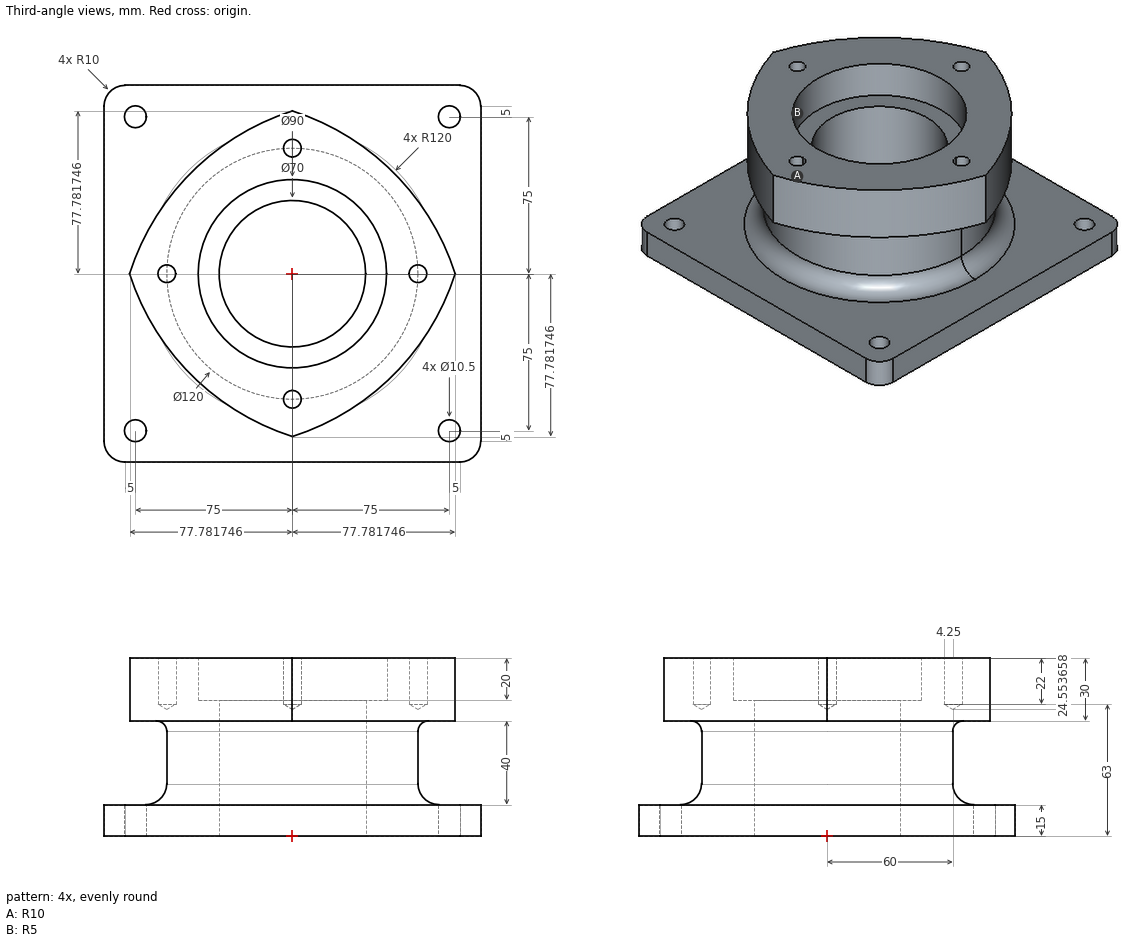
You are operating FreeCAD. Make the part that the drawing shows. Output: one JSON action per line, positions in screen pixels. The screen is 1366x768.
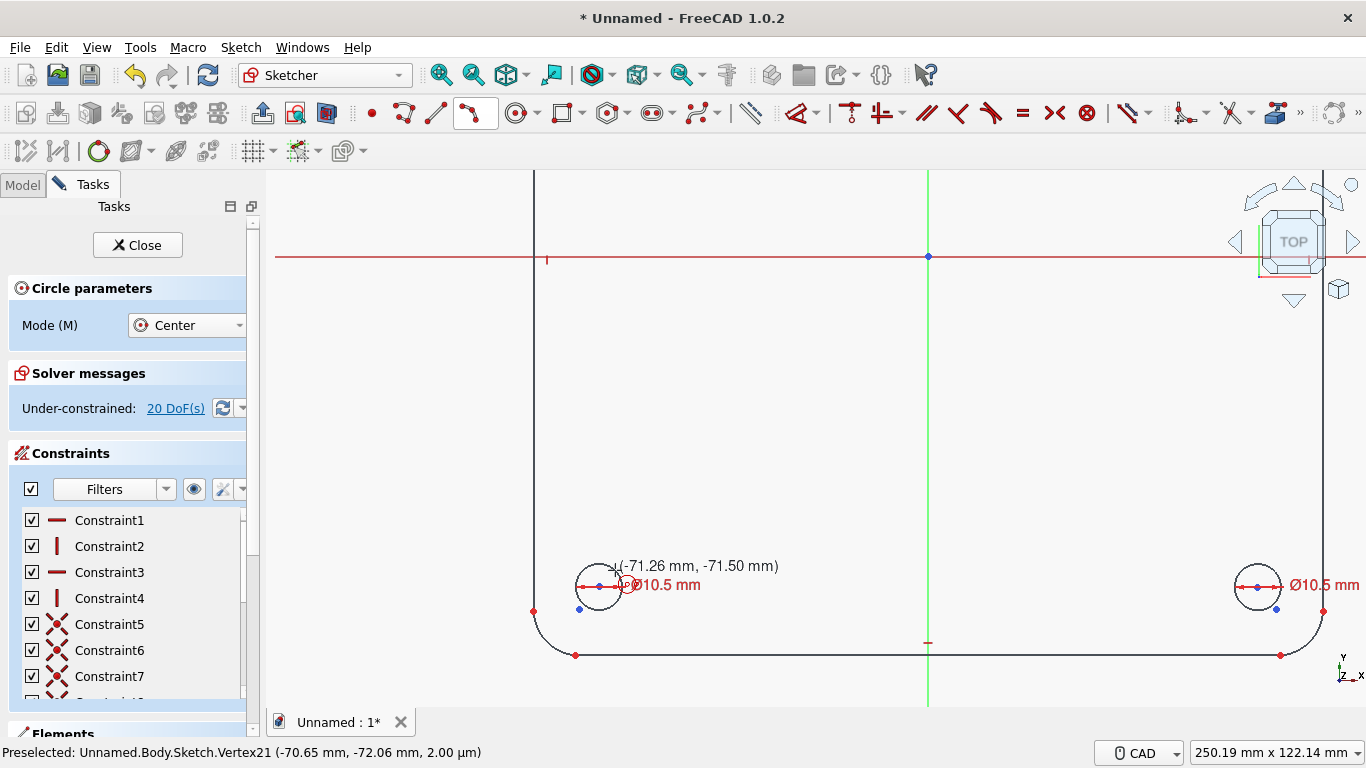
{"action": "scroll", "coordinate": [600, 587], "scroll_direction": "down", "scroll_amount": 4}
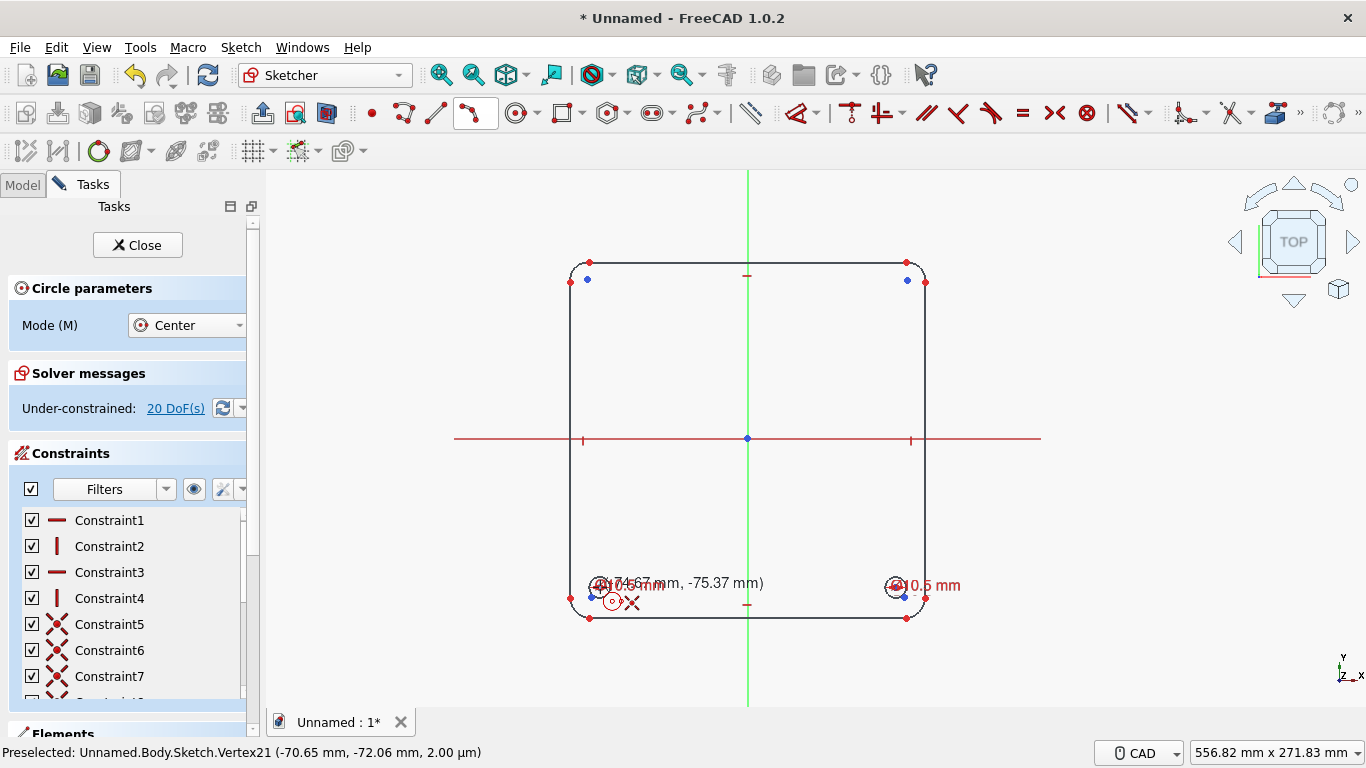
{"action": "scroll", "coordinate": [896, 291], "scroll_direction": "up", "scroll_amount": 4}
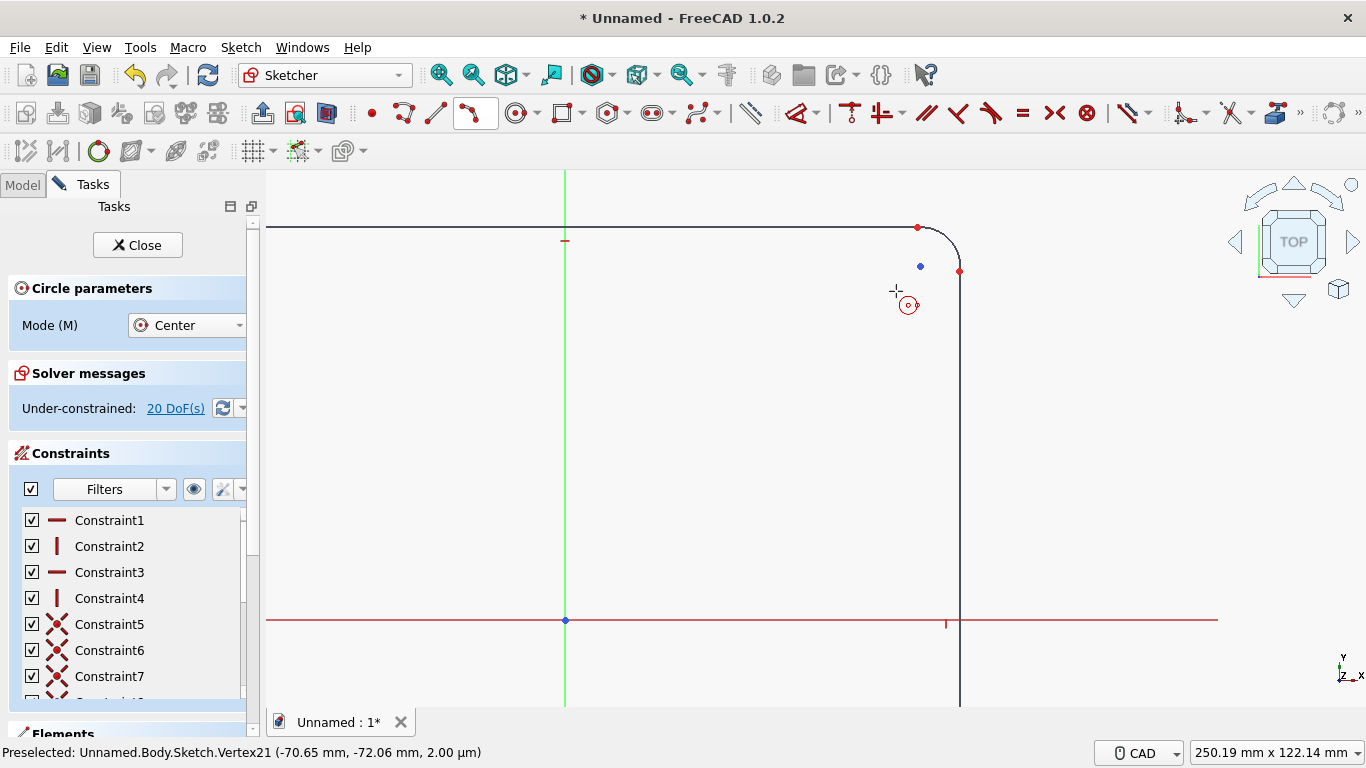
{"action": "left_click", "coordinate": [895, 290]}
{"action": "mouse_move", "coordinate": [879, 274]}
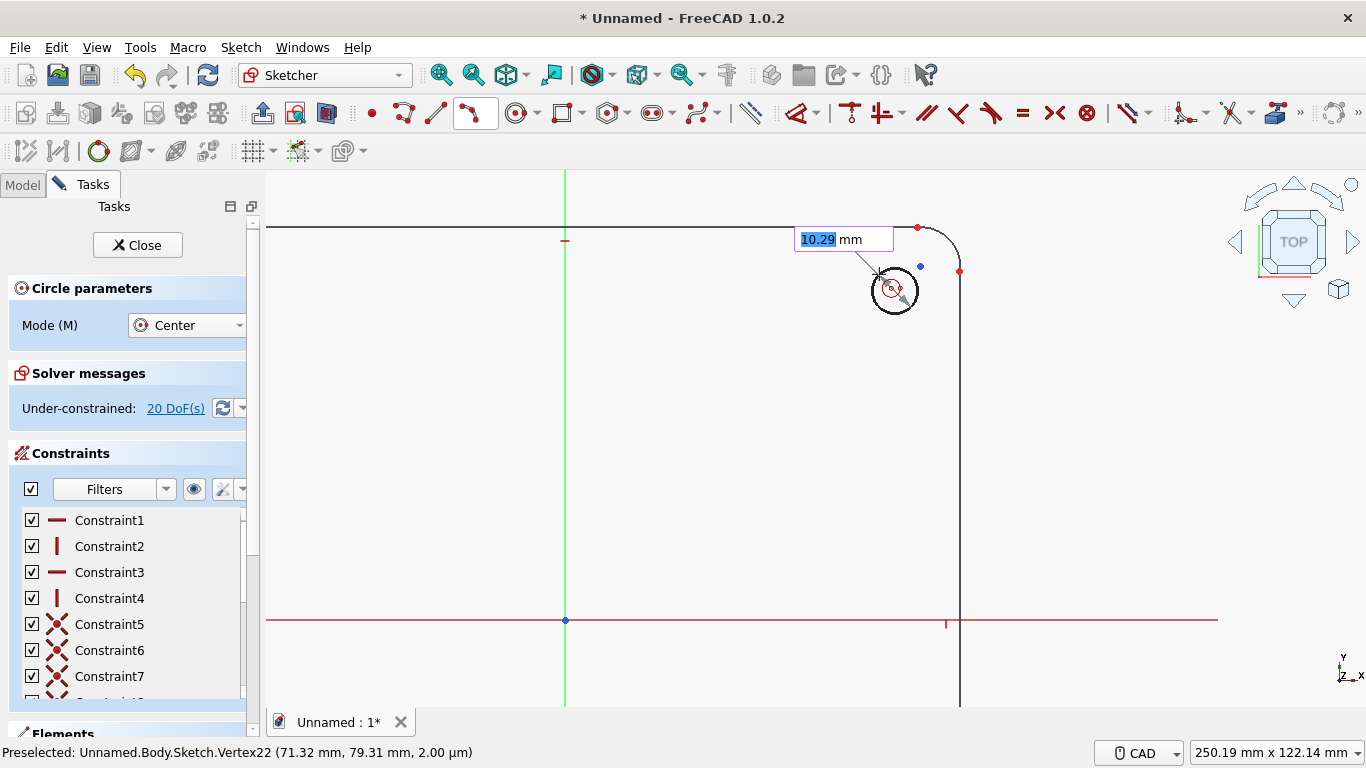
{"action": "type", "text": "10.5"}
{"action": "key", "text": "Return"}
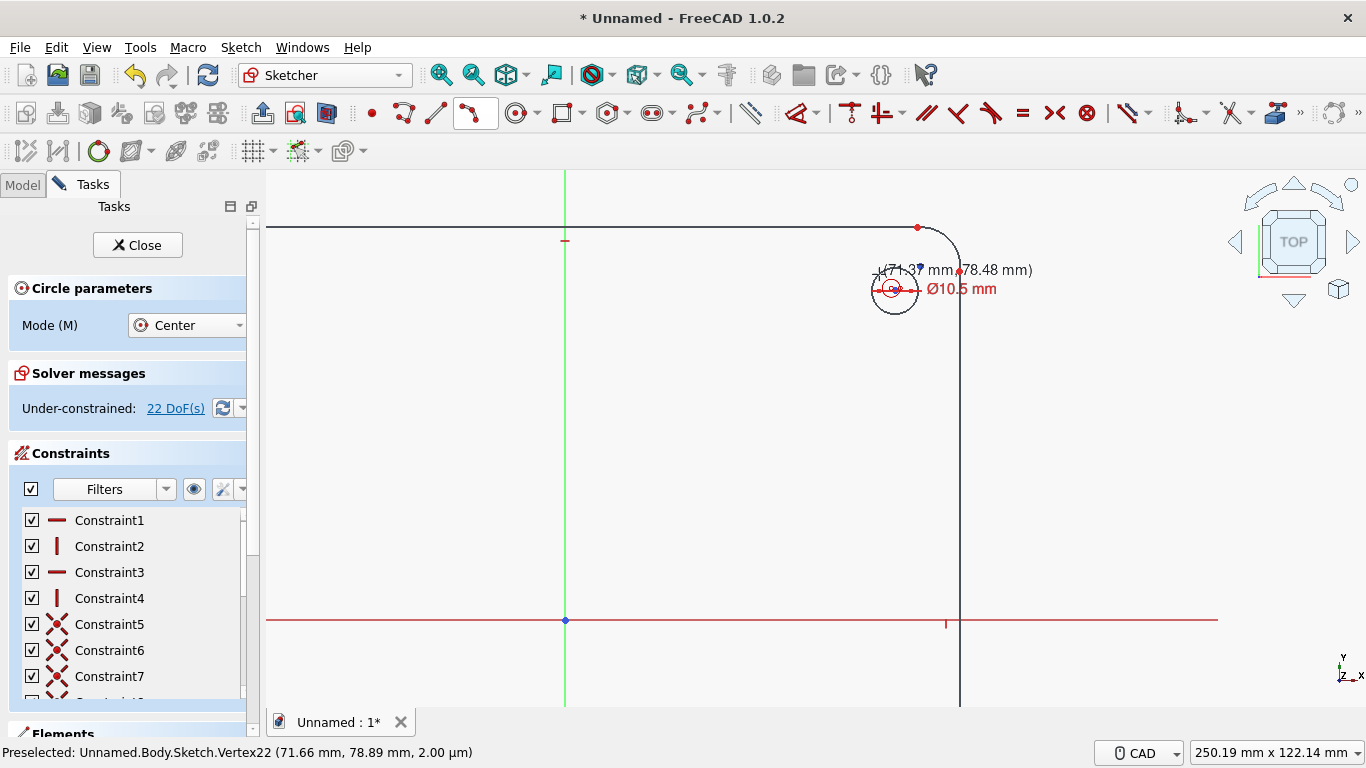
{"action": "scroll", "coordinate": [896, 290], "scroll_direction": "down", "scroll_amount": 4}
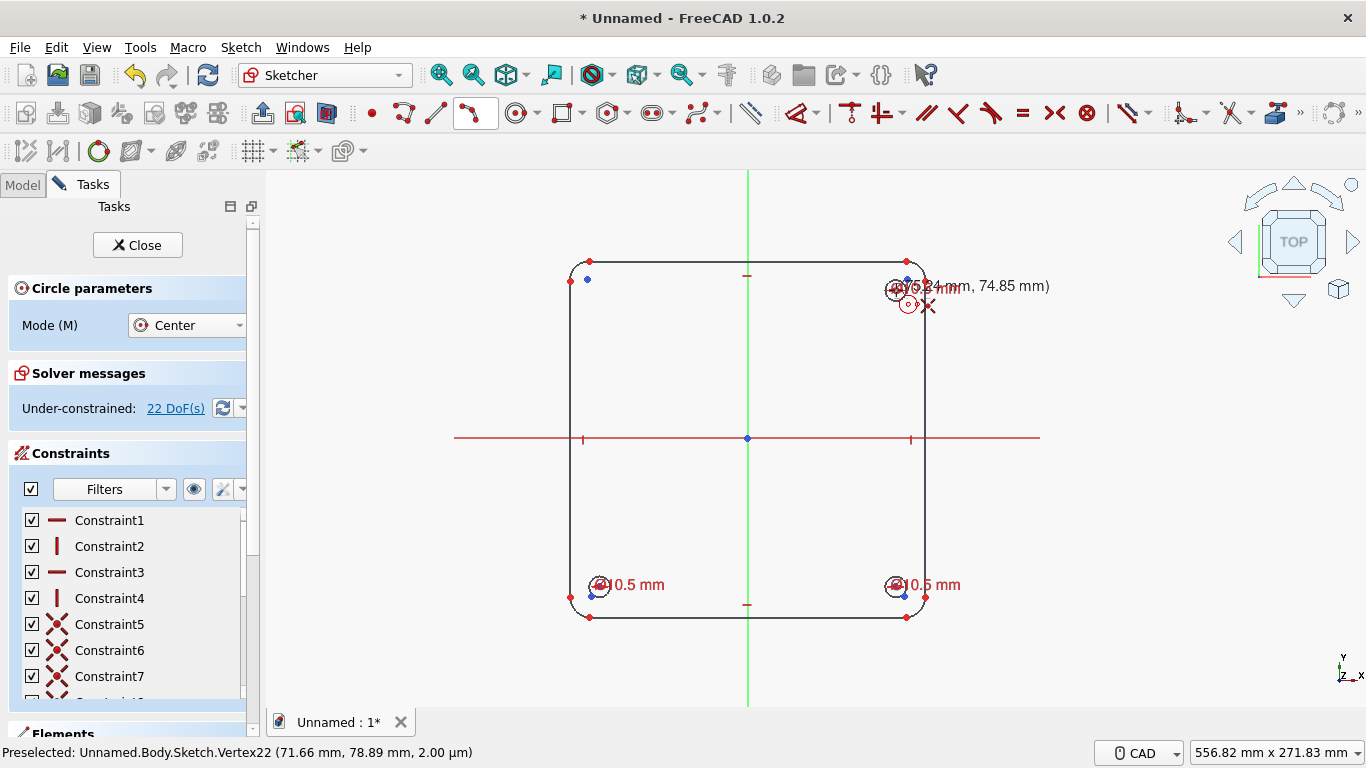
{"action": "scroll", "coordinate": [600, 290], "scroll_direction": "up", "scroll_amount": 4}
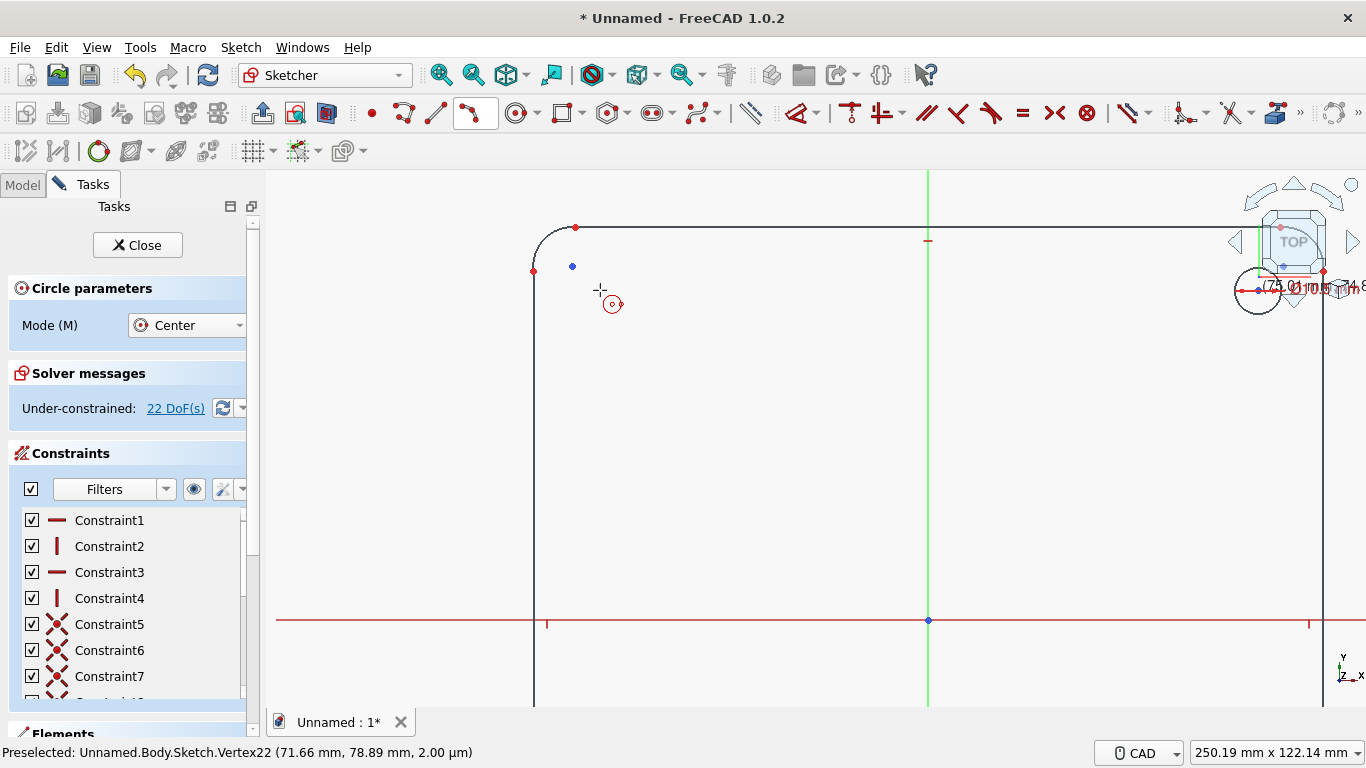
{"action": "left_click", "coordinate": [599, 290]}
{"action": "mouse_move", "coordinate": [615, 274]}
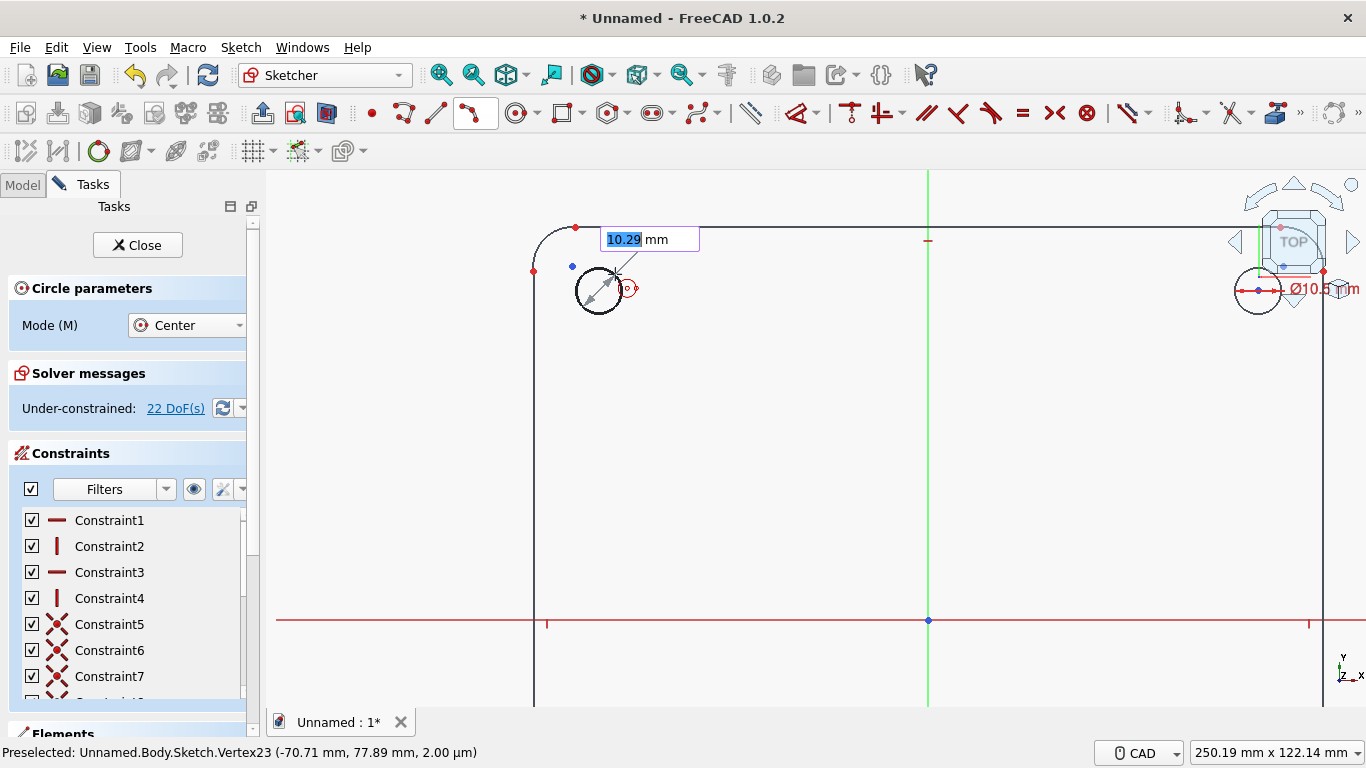
{"action": "type", "text": "10.5"}
{"action": "key", "text": "Return"}
{"action": "key", "text": "Escape"}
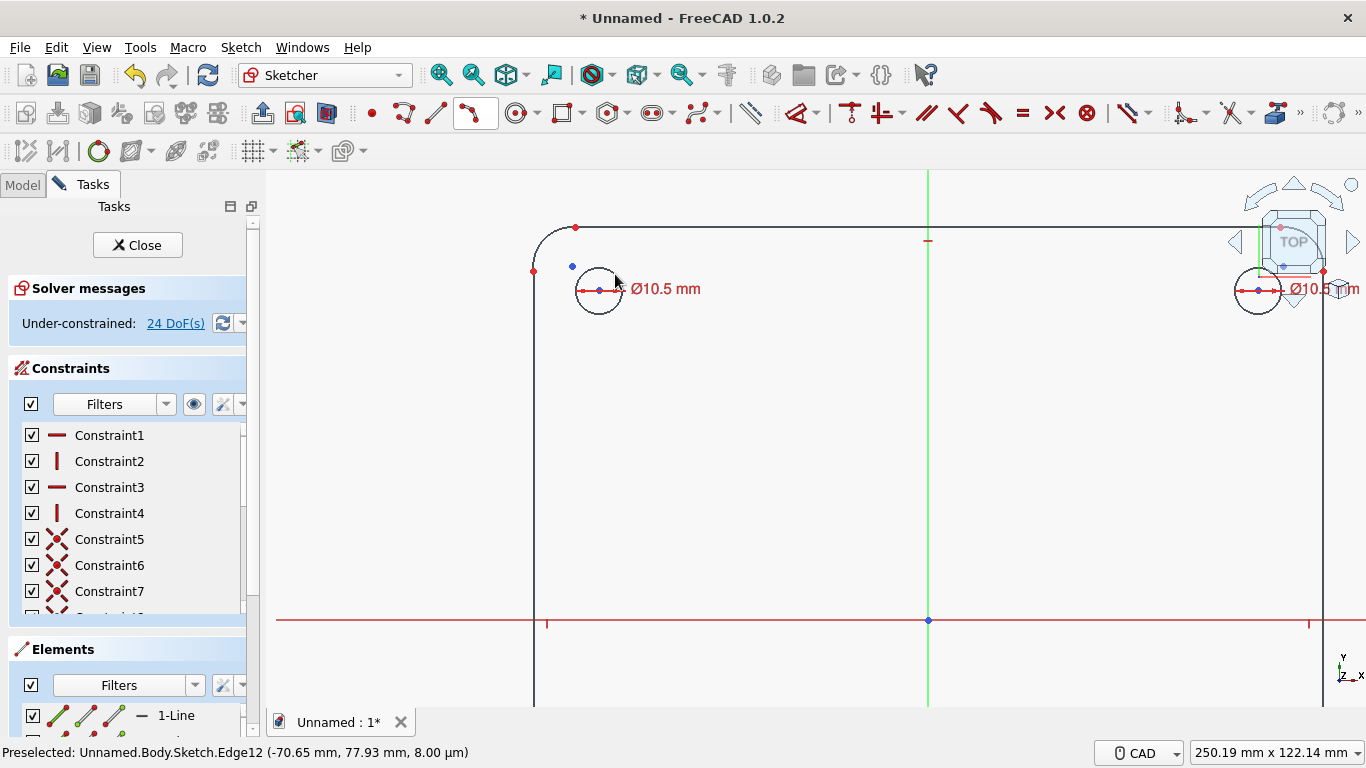
{"action": "left_click", "coordinate": [1069, 227]}